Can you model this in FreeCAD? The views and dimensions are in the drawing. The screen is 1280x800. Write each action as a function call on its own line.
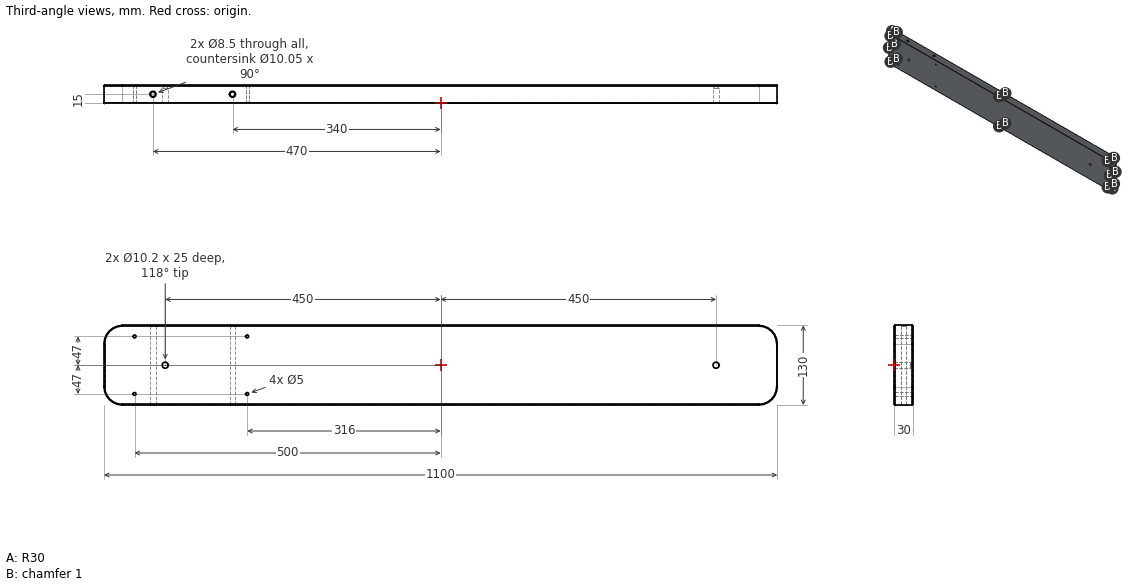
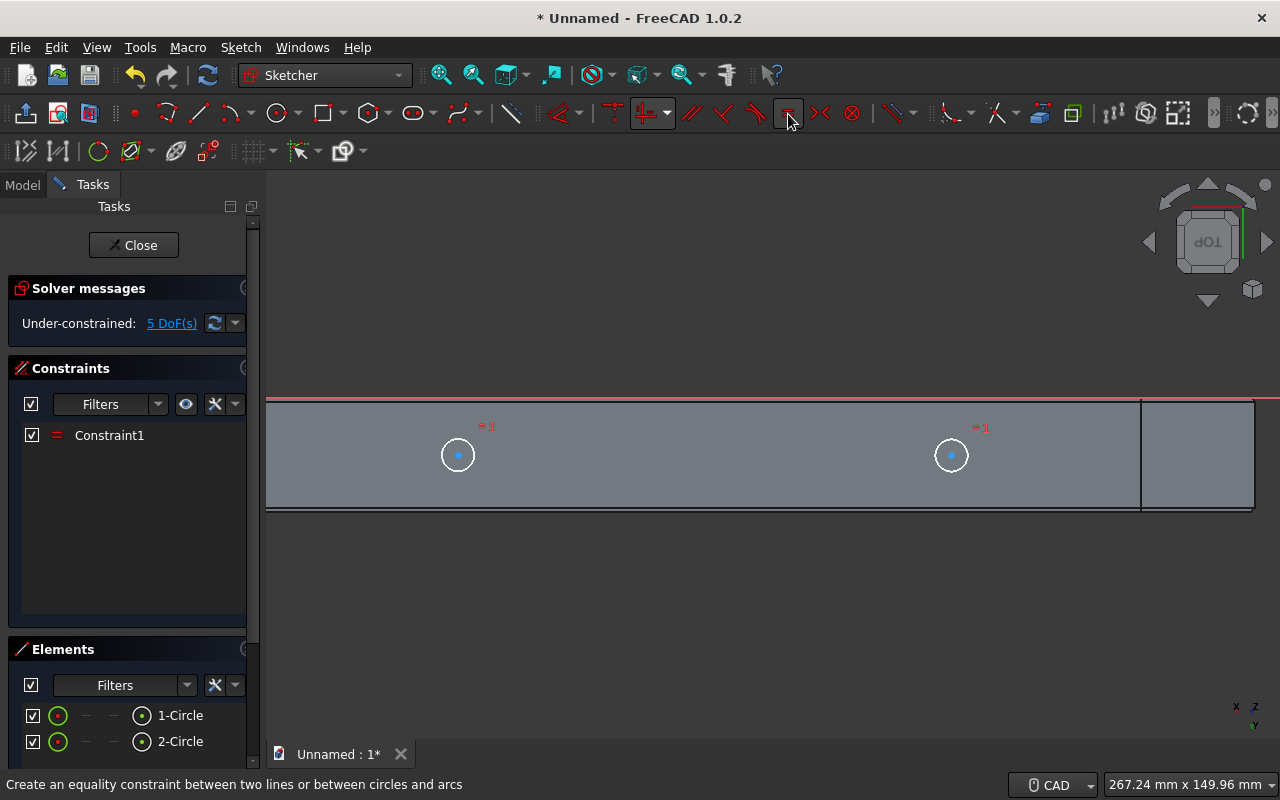
click(952, 455)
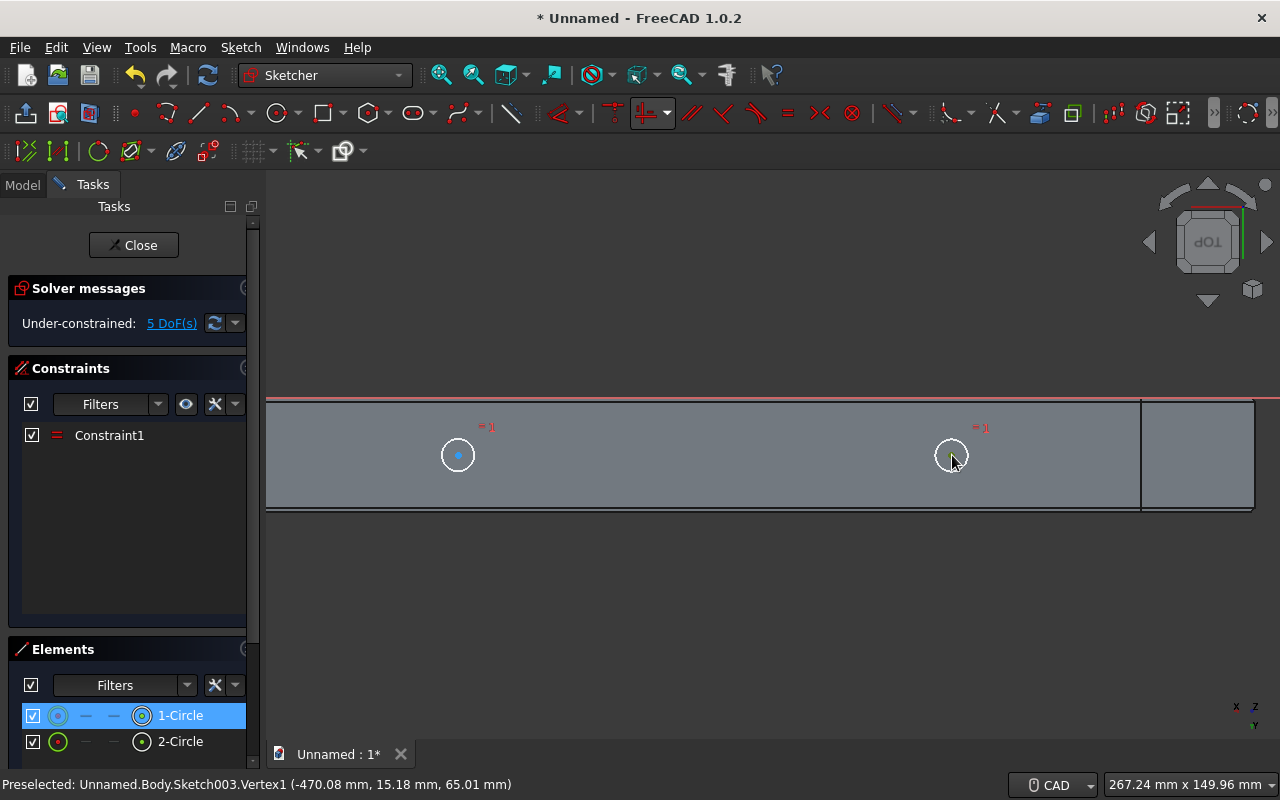
click(458, 455)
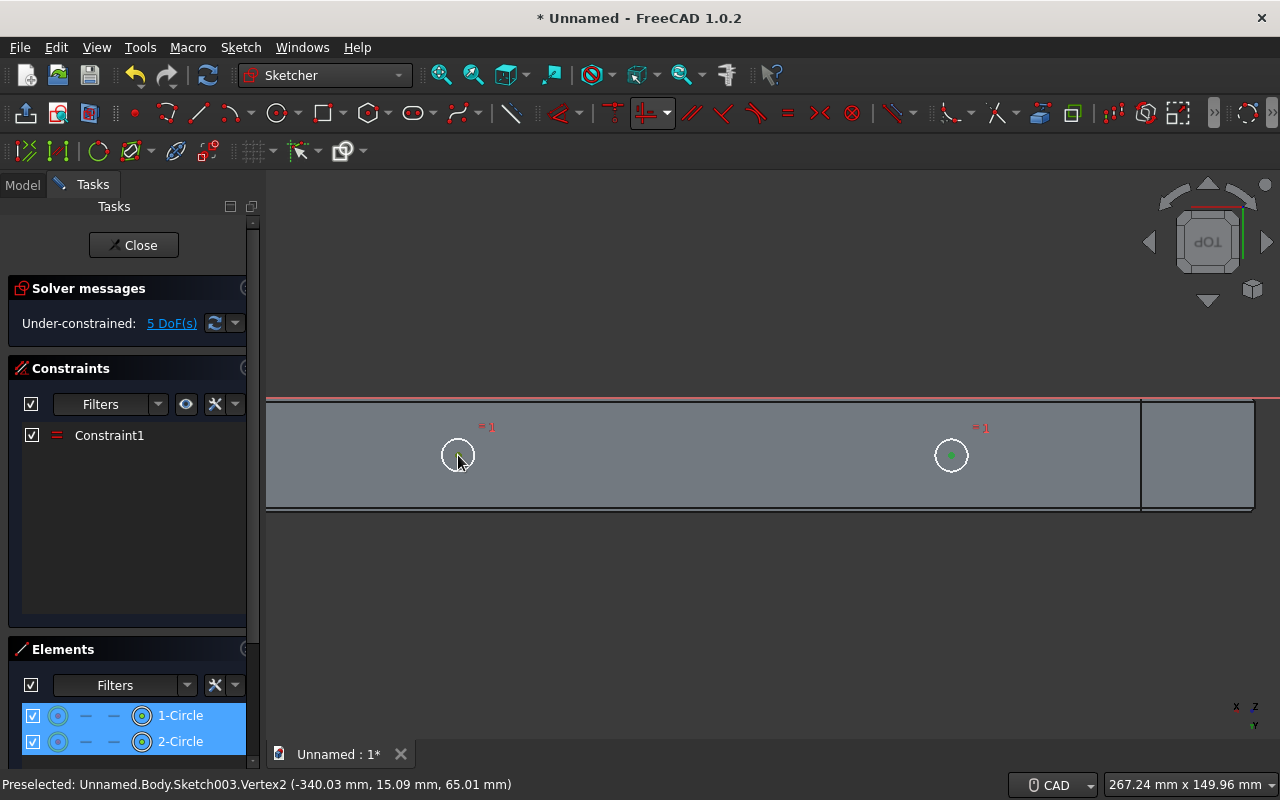
key(h)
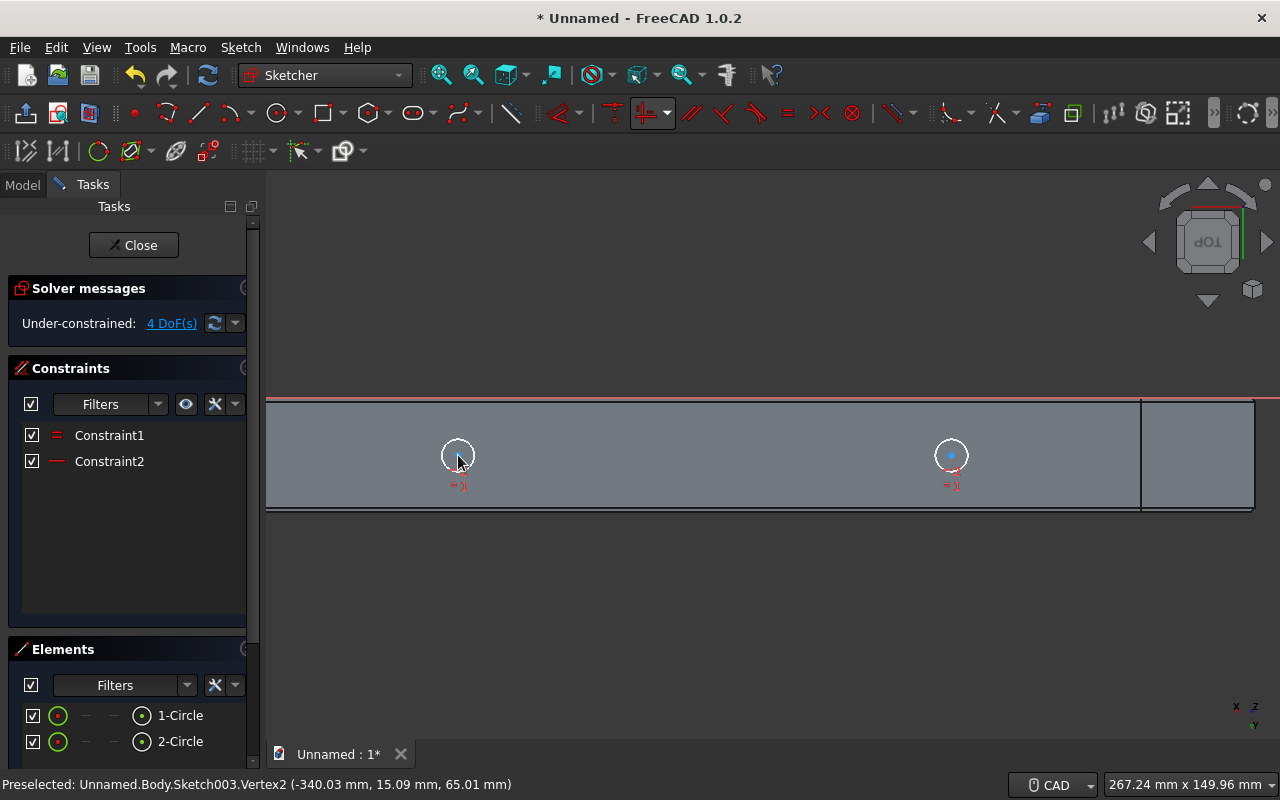
click(558, 114)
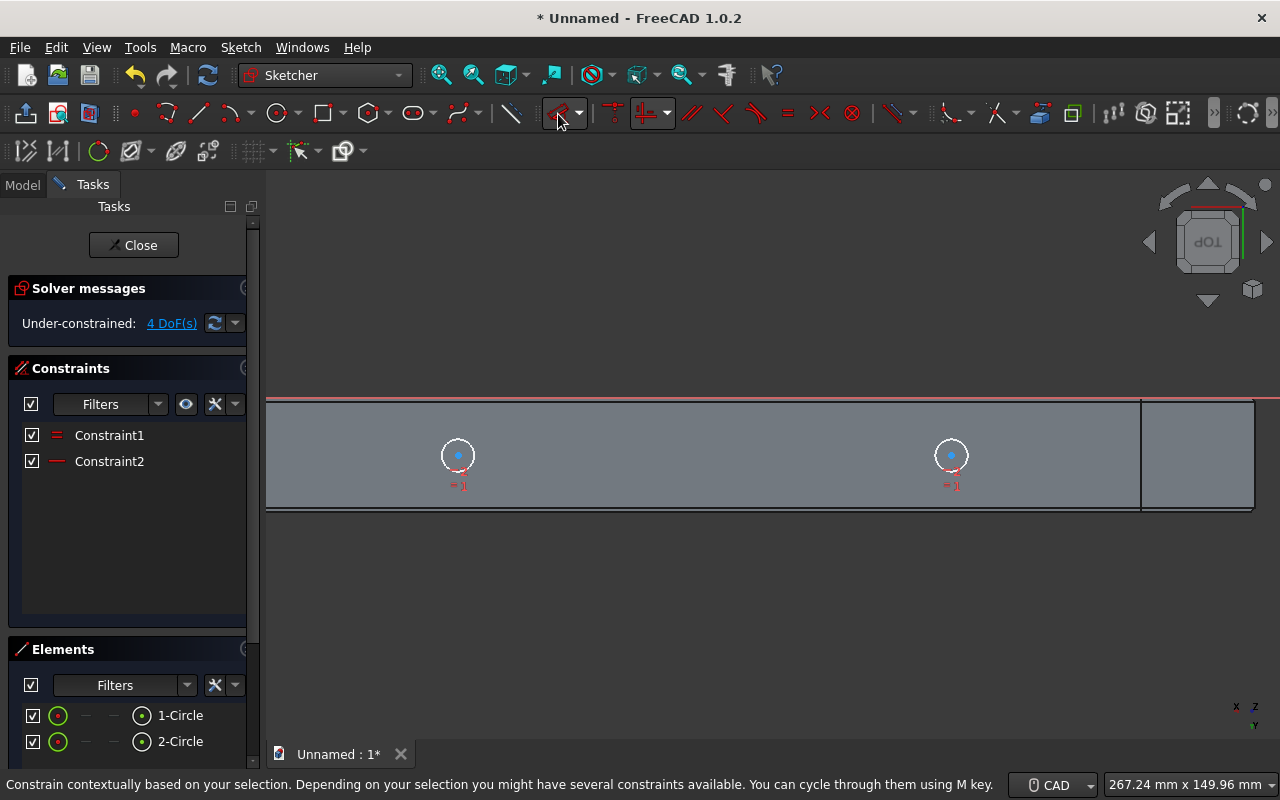
scroll(963, 444, up, 2)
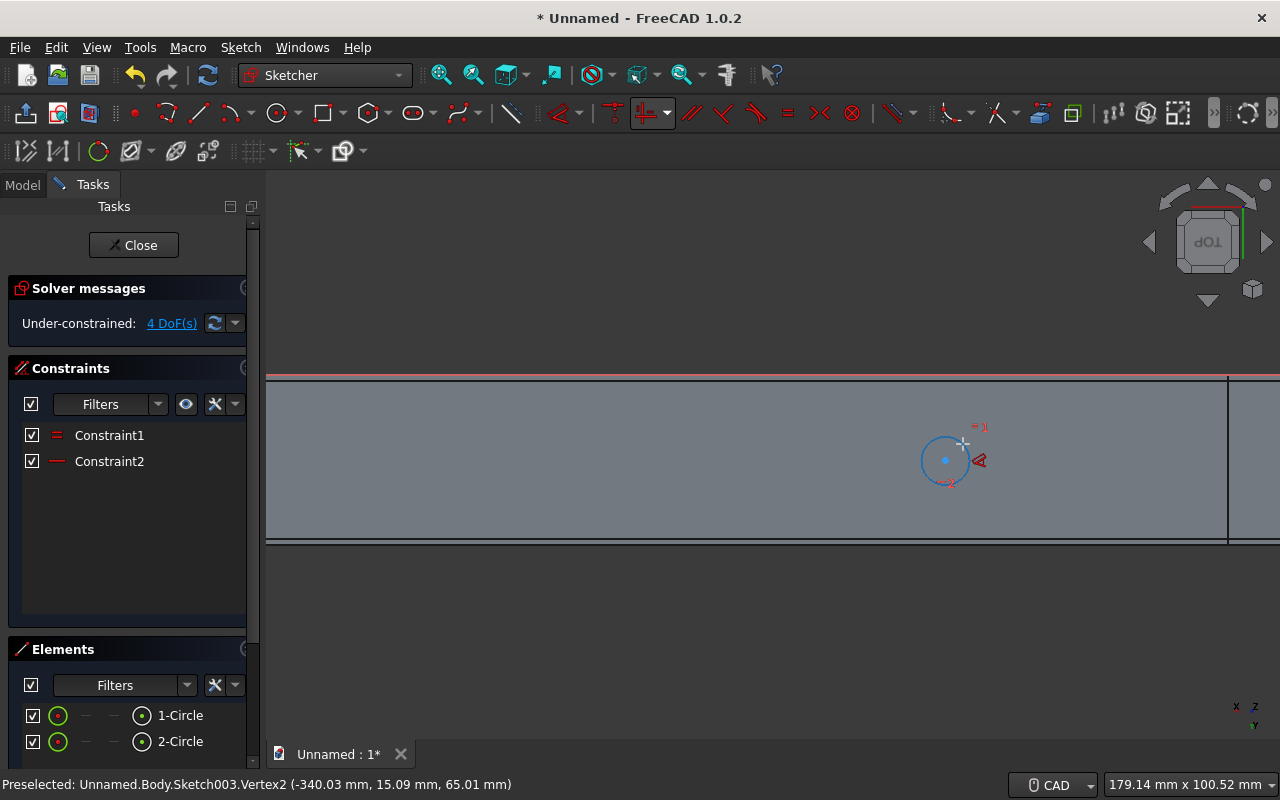
click(962, 444)
click(984, 421)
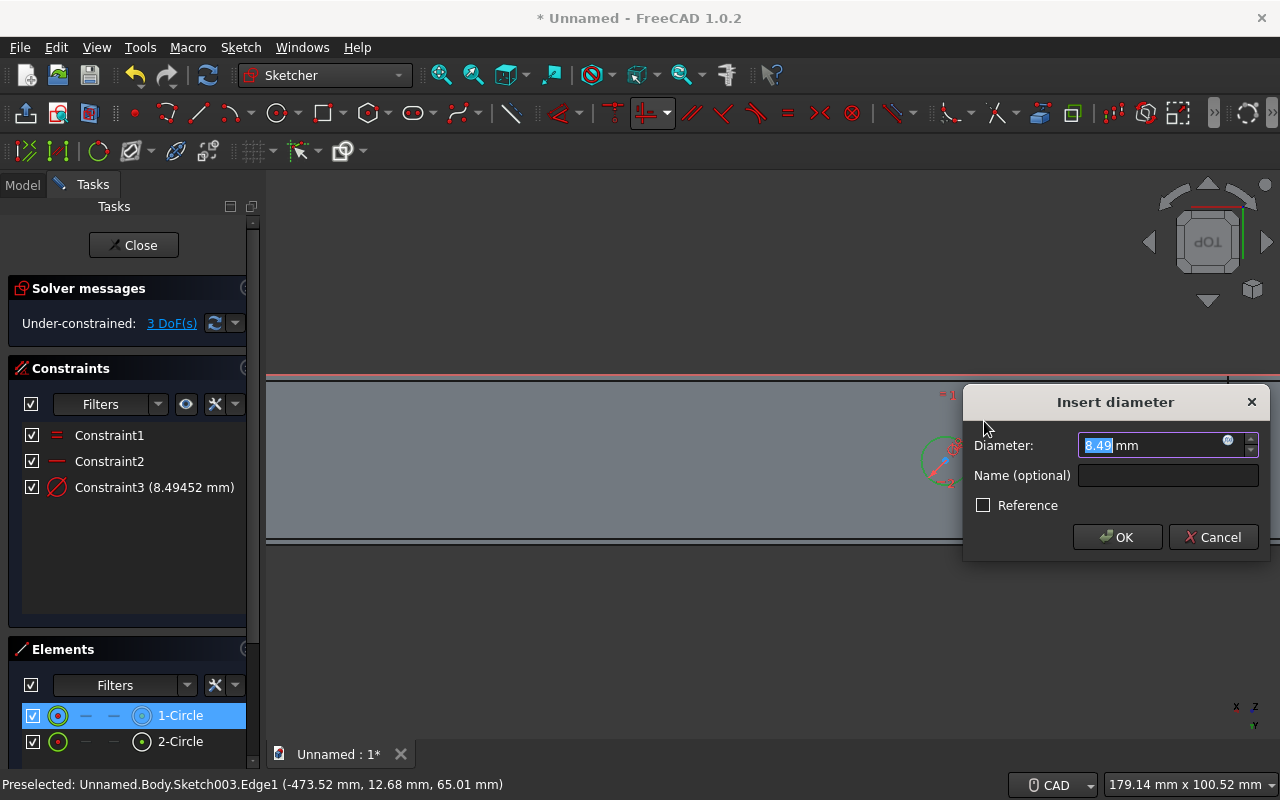
text(8.5)
key(Return)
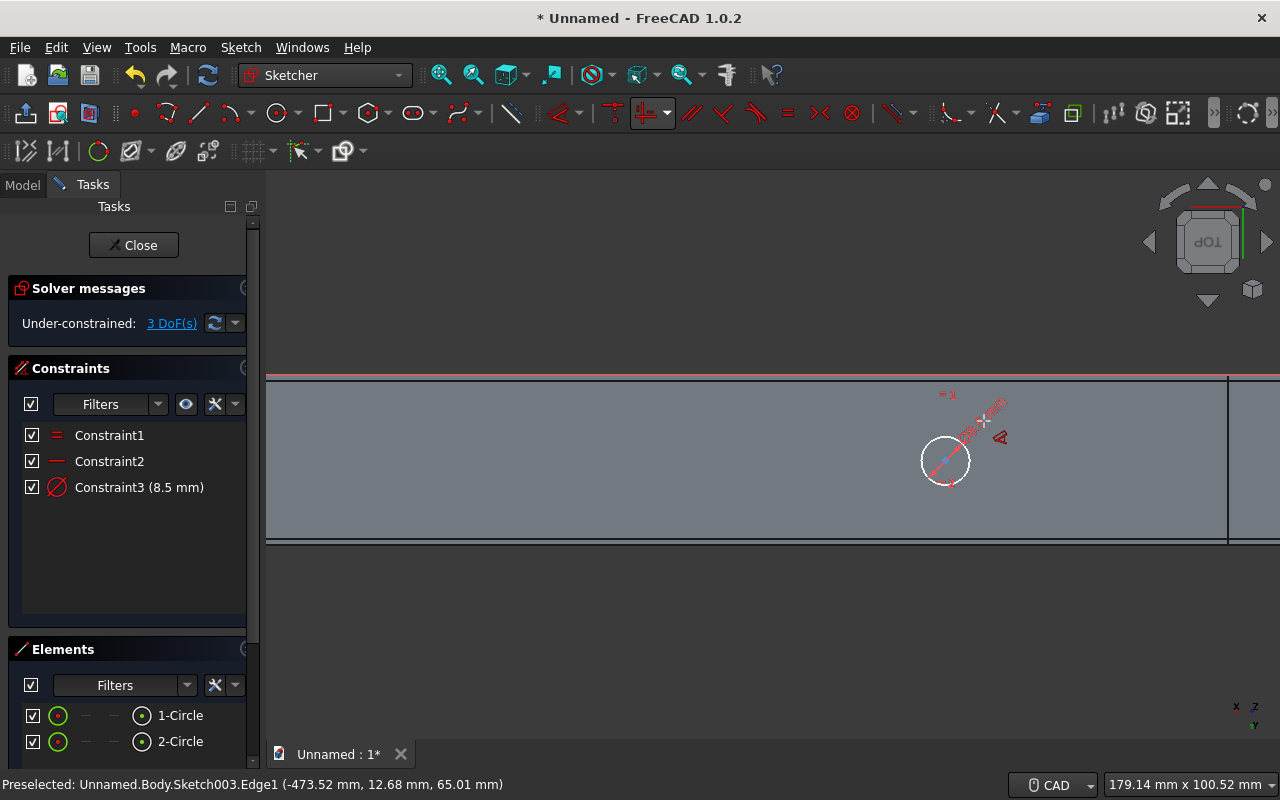
click(946, 461)
click(980, 398)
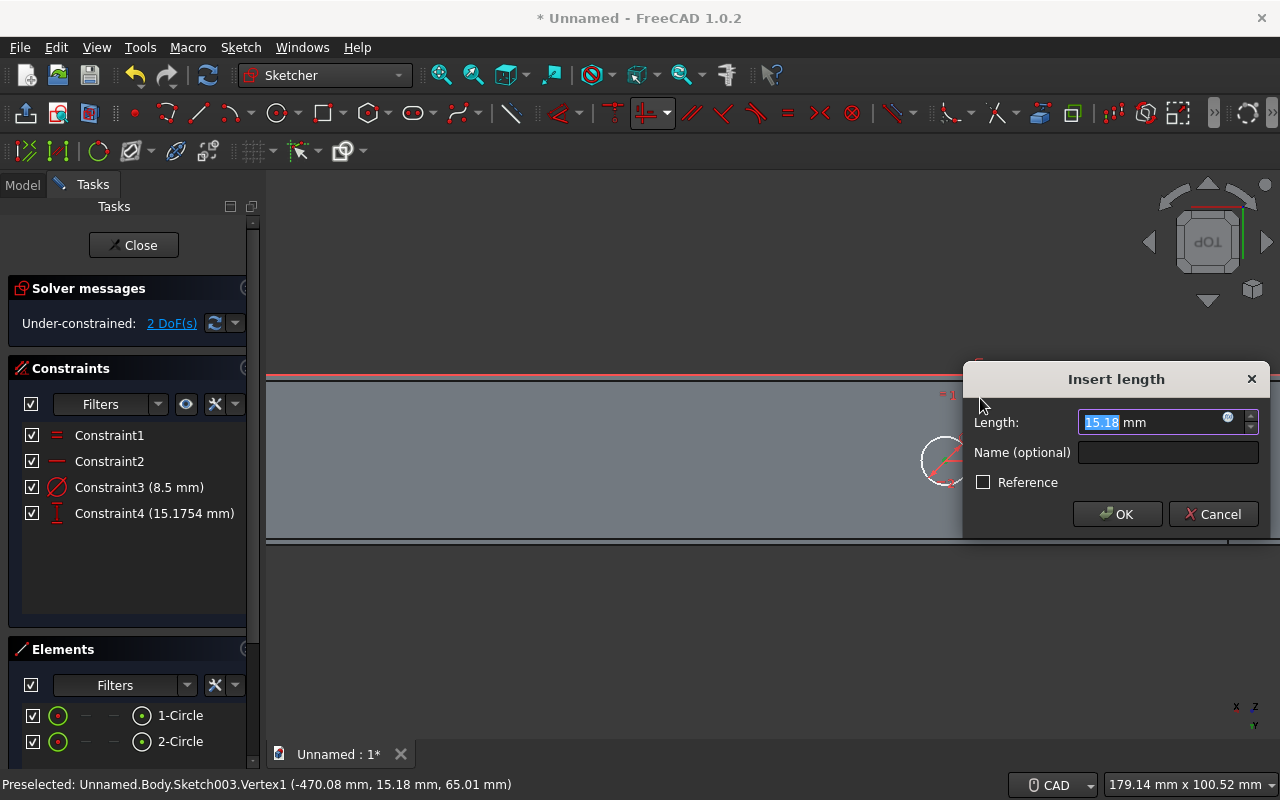
text(15)
key(Return)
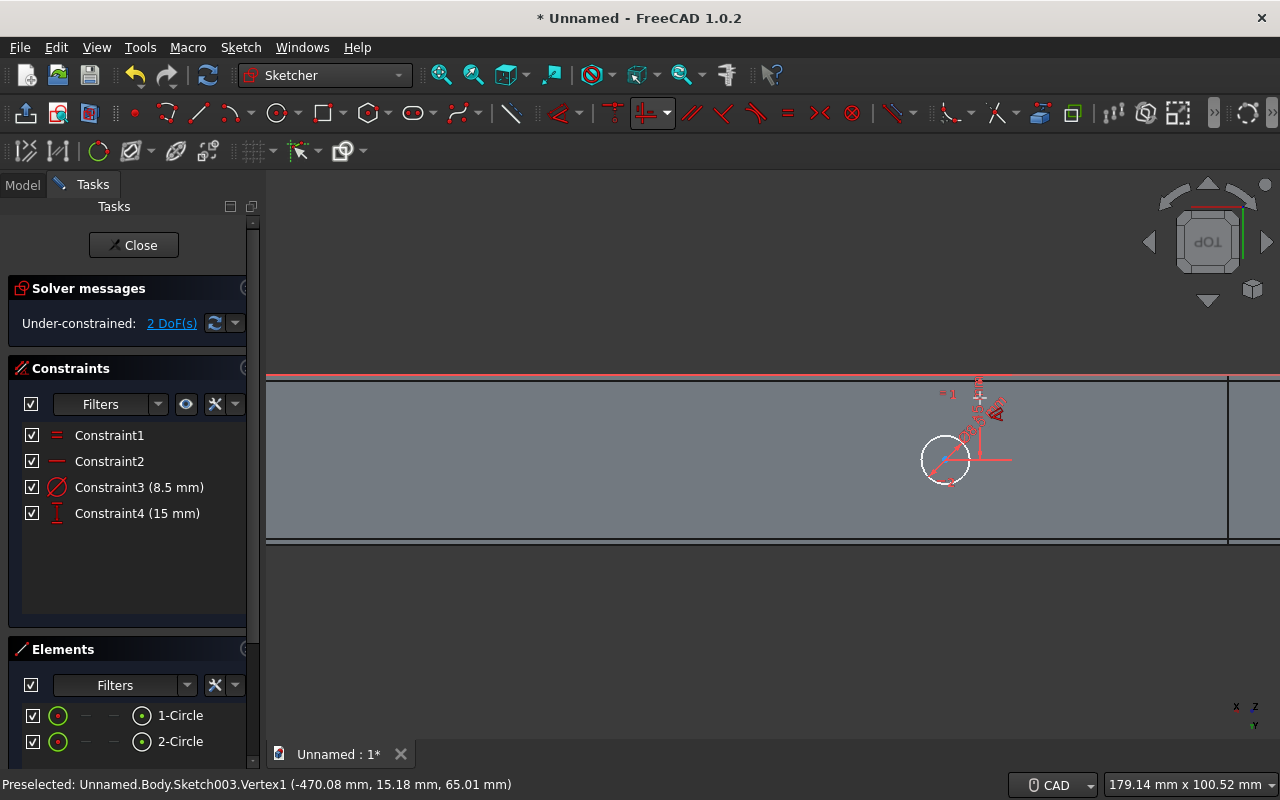
click(946, 460)
click(620, 341)